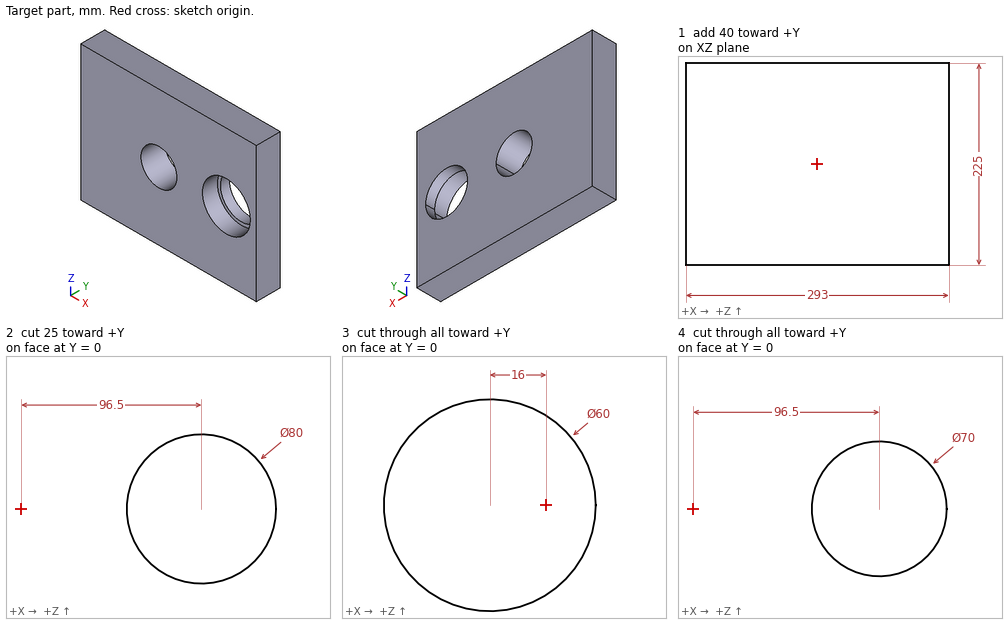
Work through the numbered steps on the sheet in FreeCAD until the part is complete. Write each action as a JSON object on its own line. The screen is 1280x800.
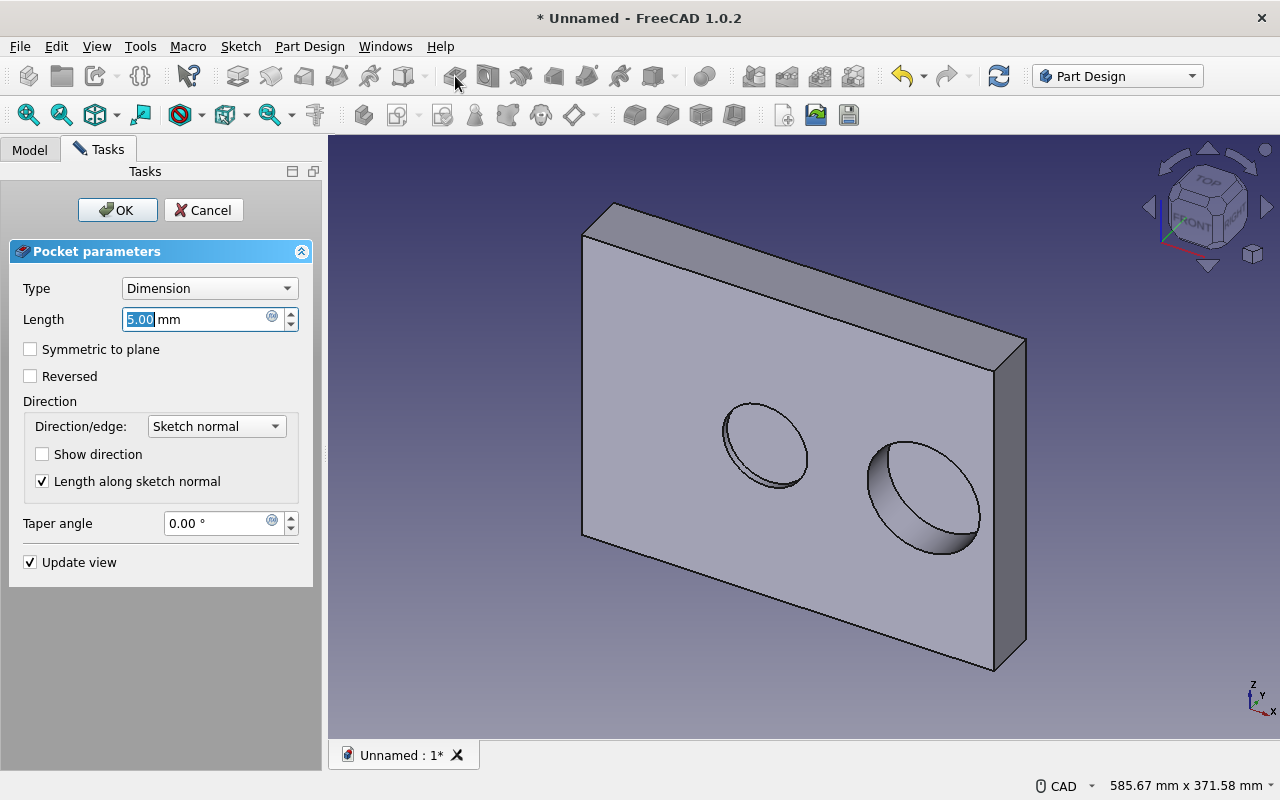
{"action": "left_click", "coordinate": [210, 288]}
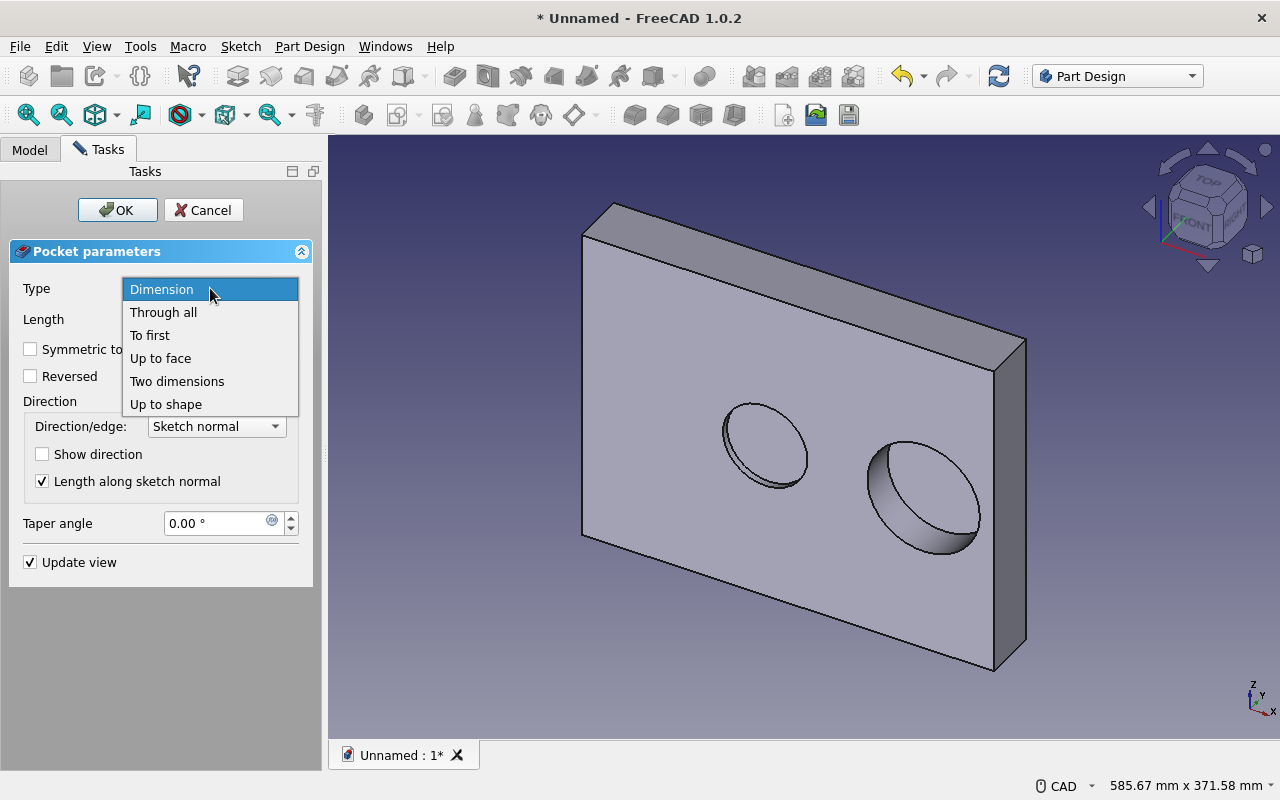
{"action": "left_click", "coordinate": [208, 312]}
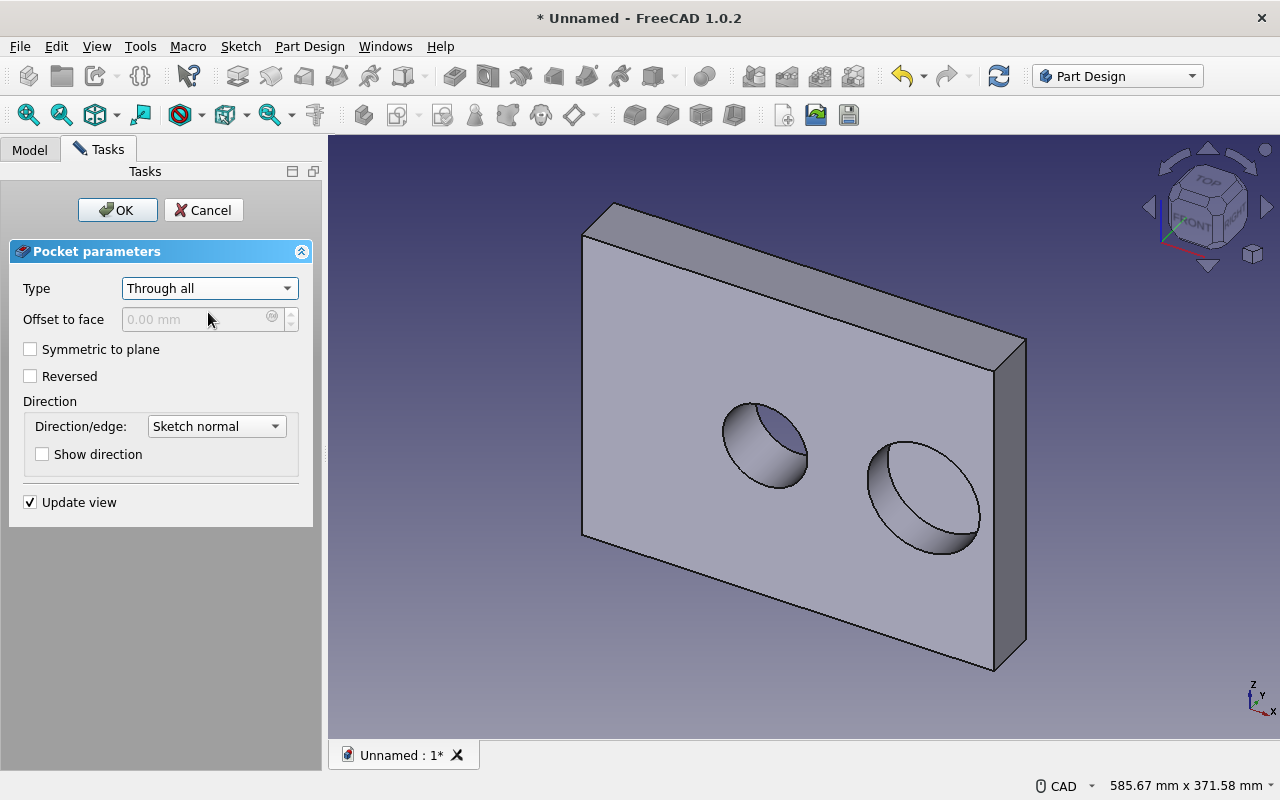
{"action": "left_click", "coordinate": [118, 210]}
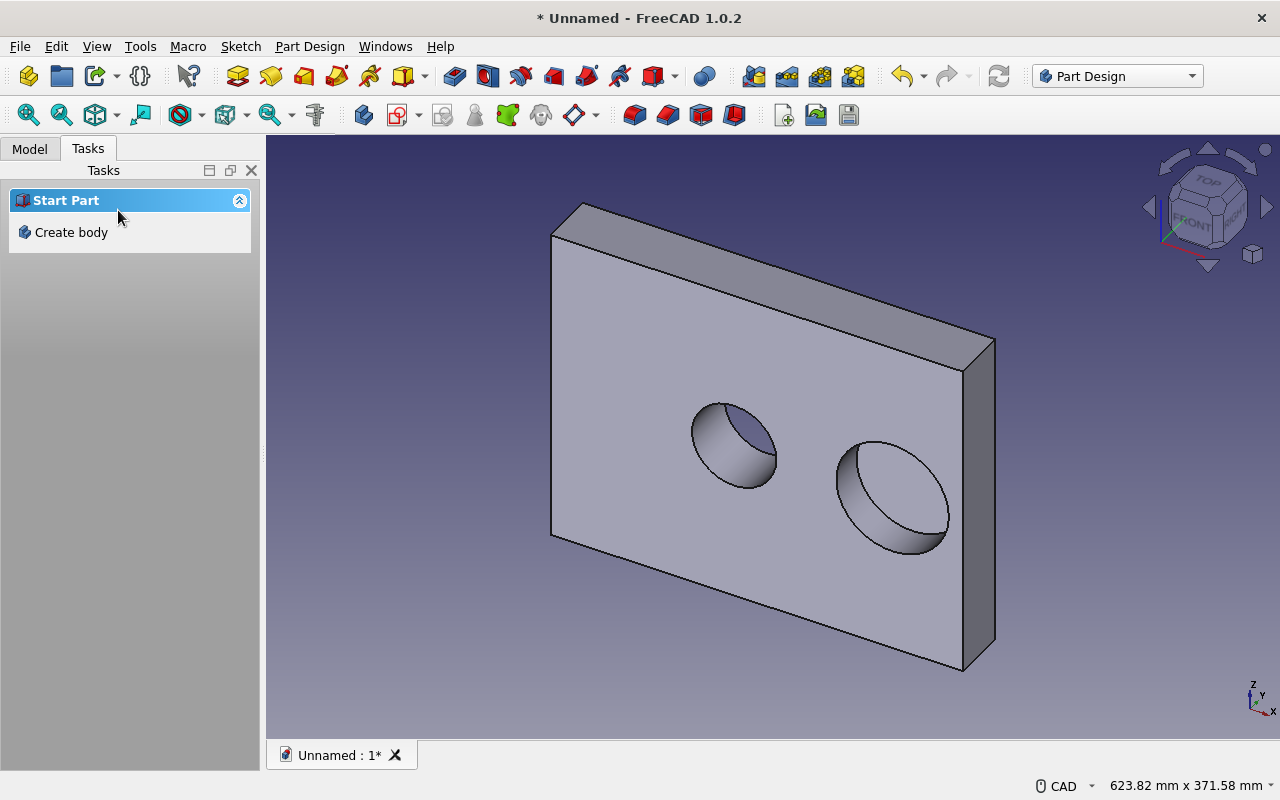
{"action": "left_click", "coordinate": [639, 328]}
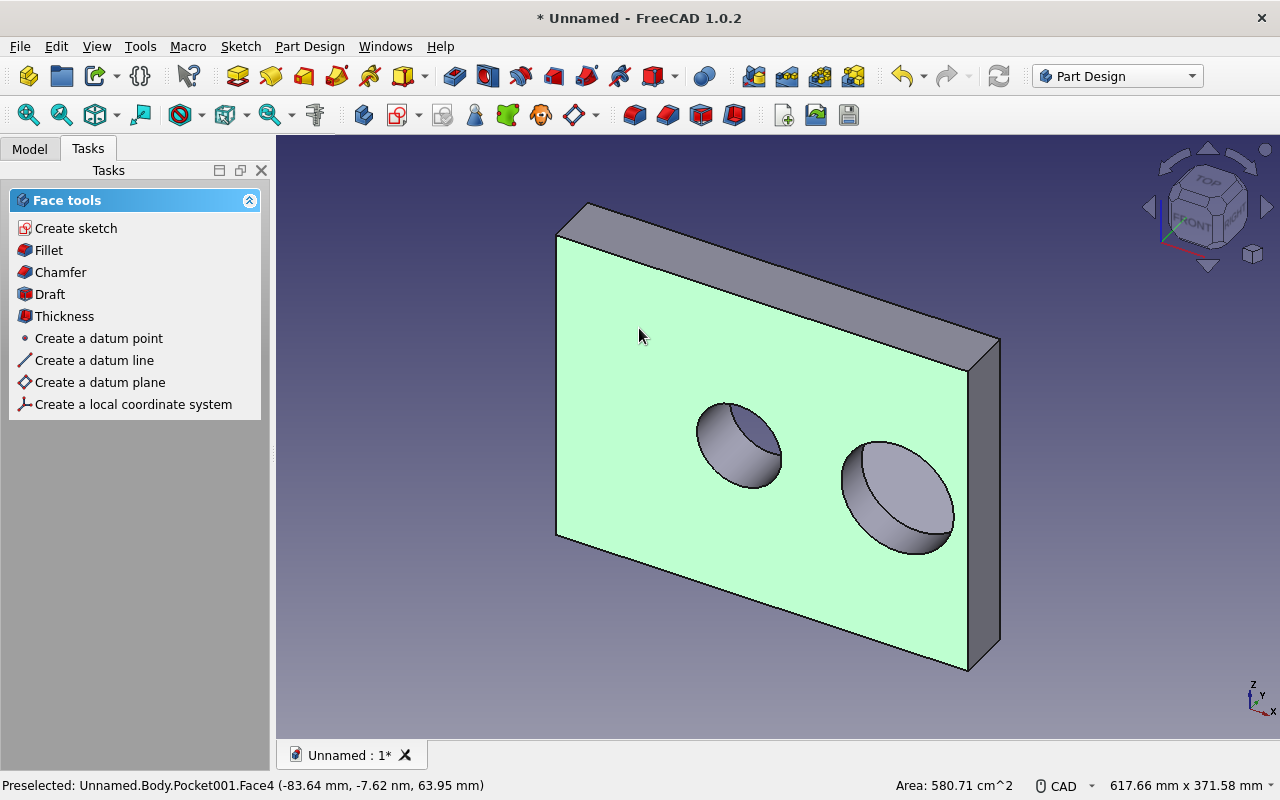
{"action": "left_click", "coordinate": [396, 116]}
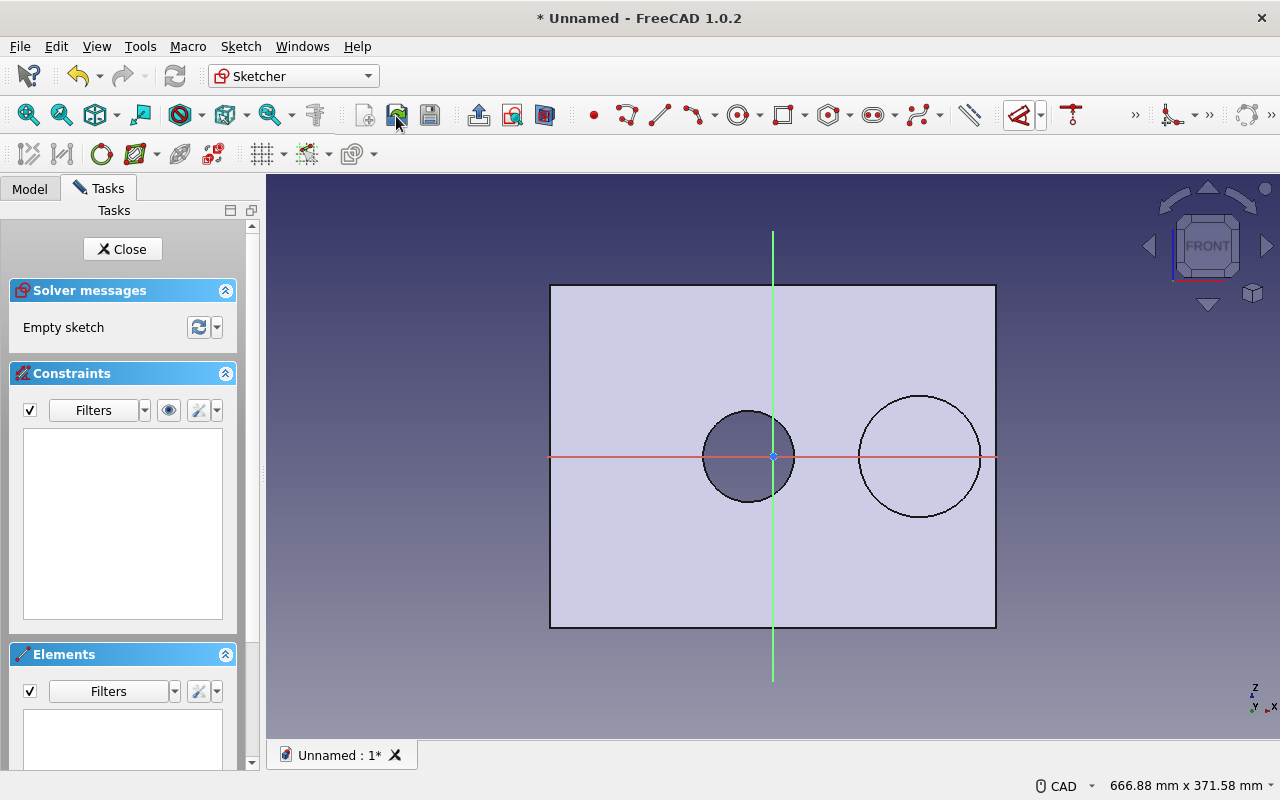
{"action": "scroll", "coordinate": [971, 457], "scroll_direction": "up", "scroll_amount": 5}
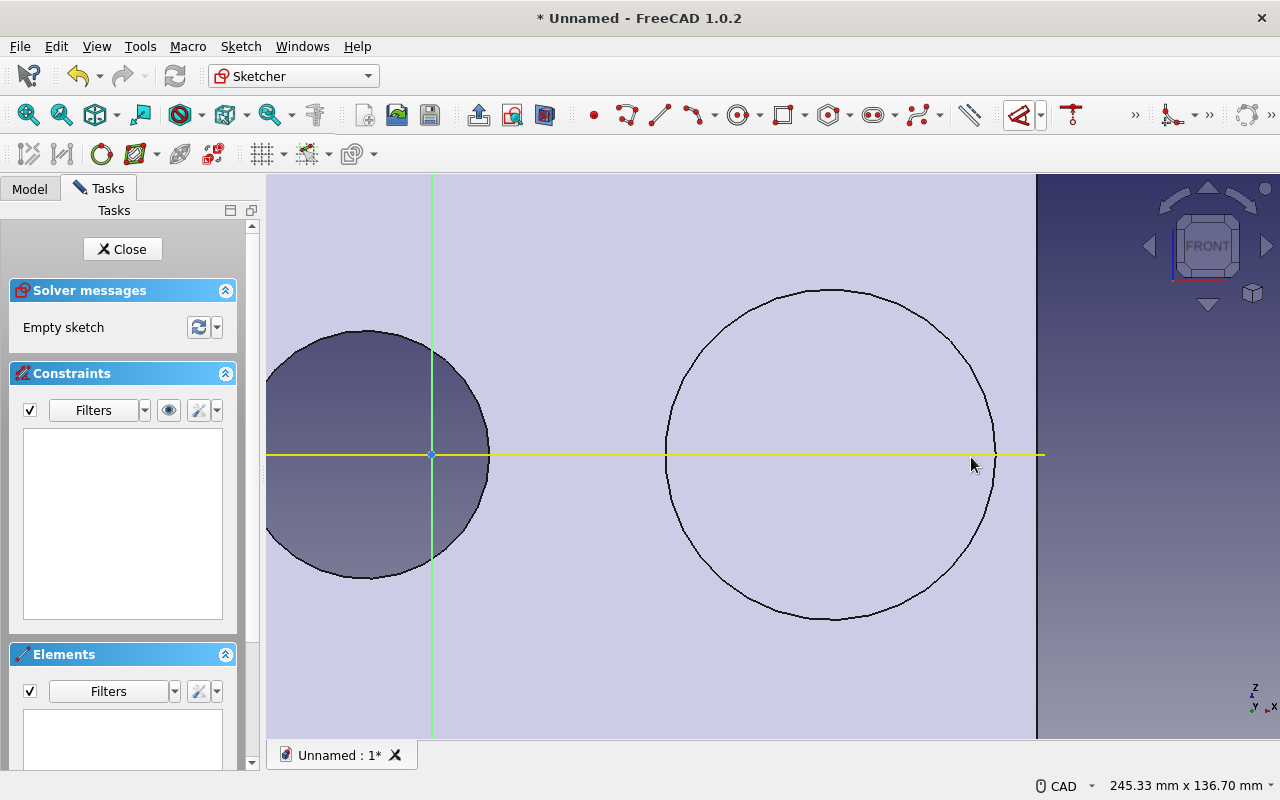
{"action": "key", "text": "g c"}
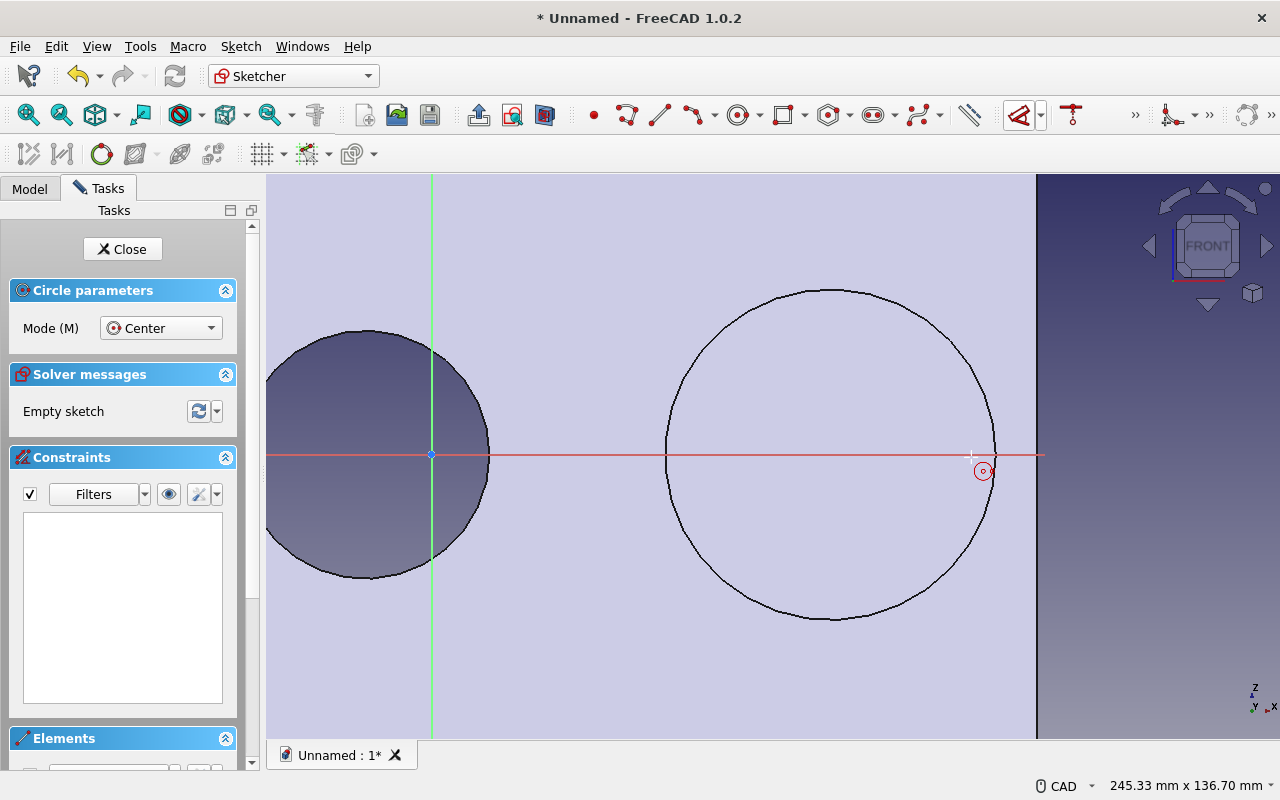
{"action": "left_click", "coordinate": [830, 455]}
{"action": "mouse_move", "coordinate": [933, 352]}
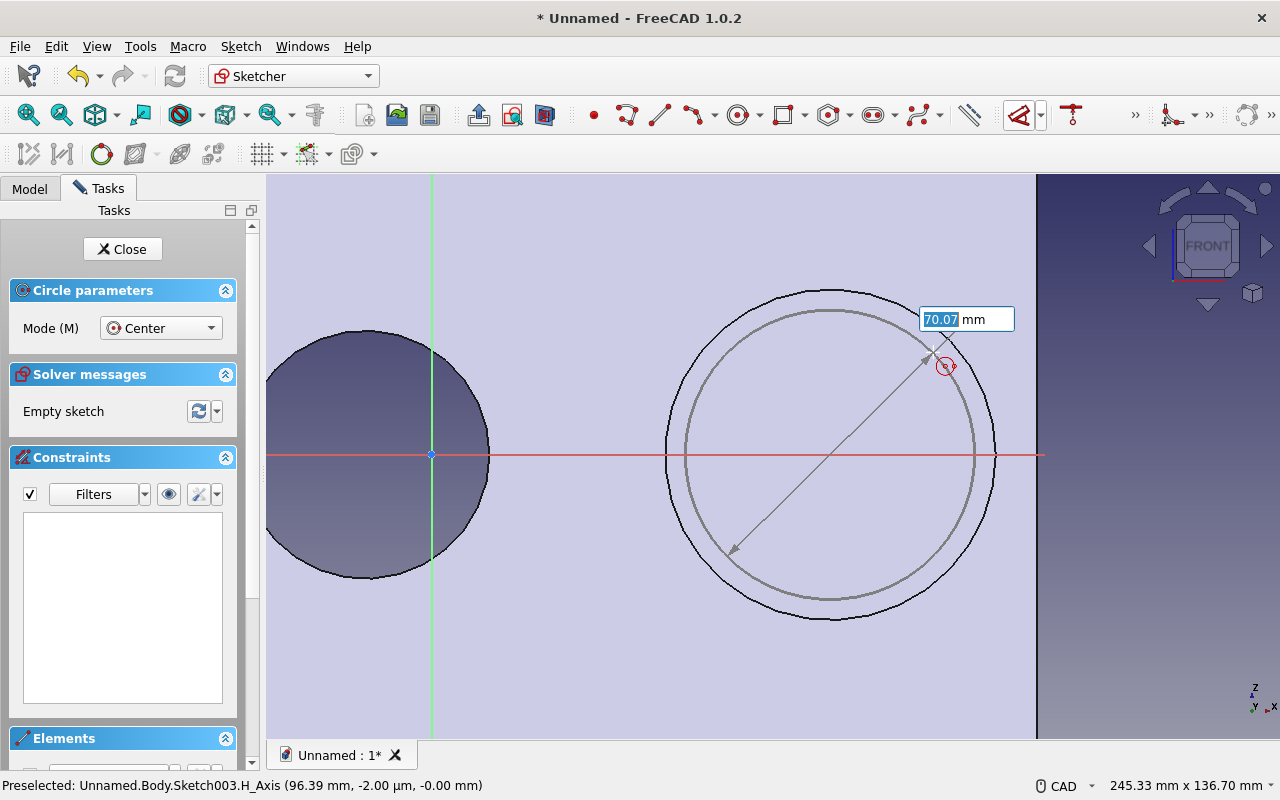
{"action": "type", "text": "70"}
{"action": "key", "text": "Return"}
{"action": "key", "text": "Escape"}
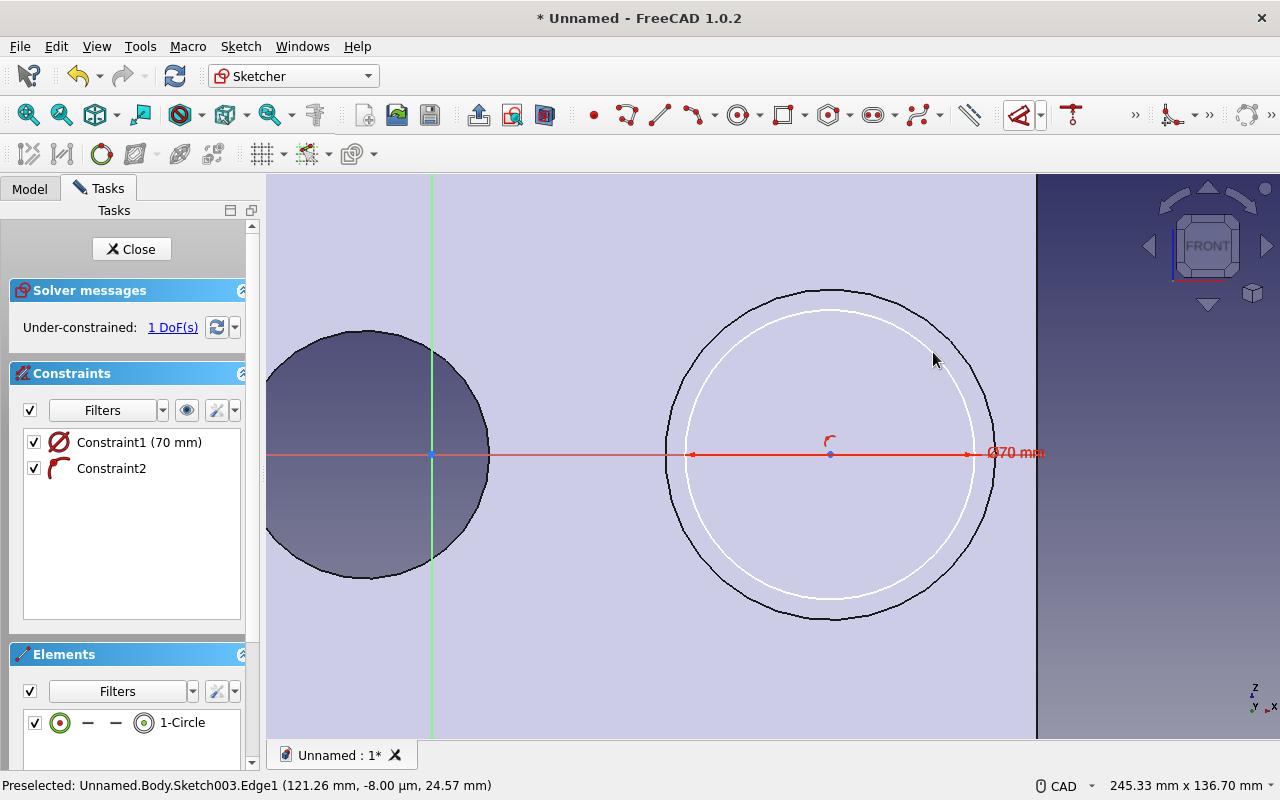
{"action": "left_click", "coordinate": [830, 455]}